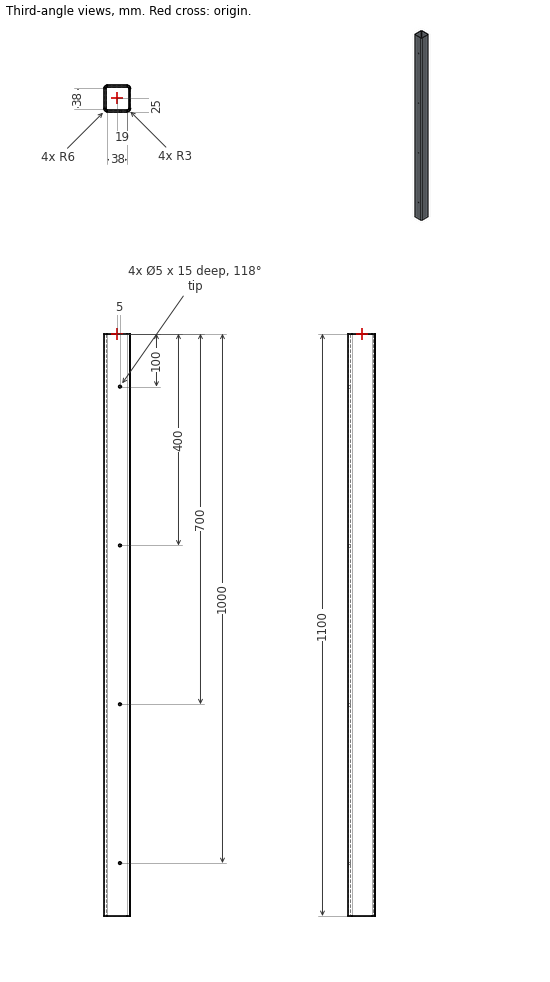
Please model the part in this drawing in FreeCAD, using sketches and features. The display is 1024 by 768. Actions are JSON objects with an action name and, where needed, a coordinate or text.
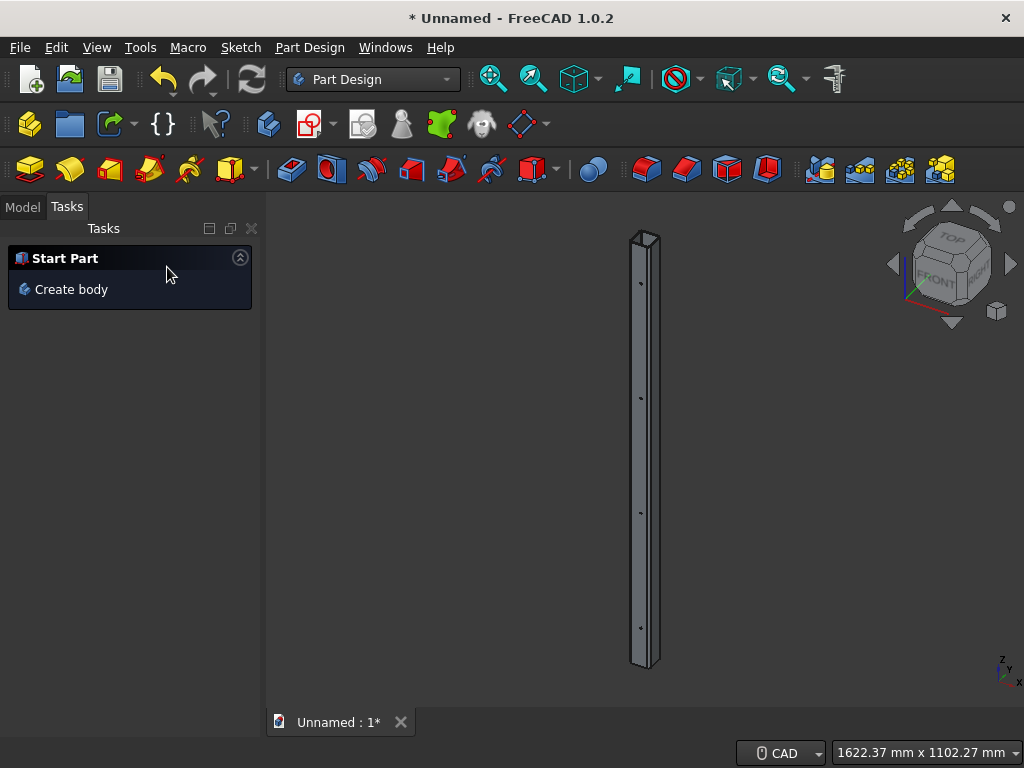
{"action": "key", "text": "0"}